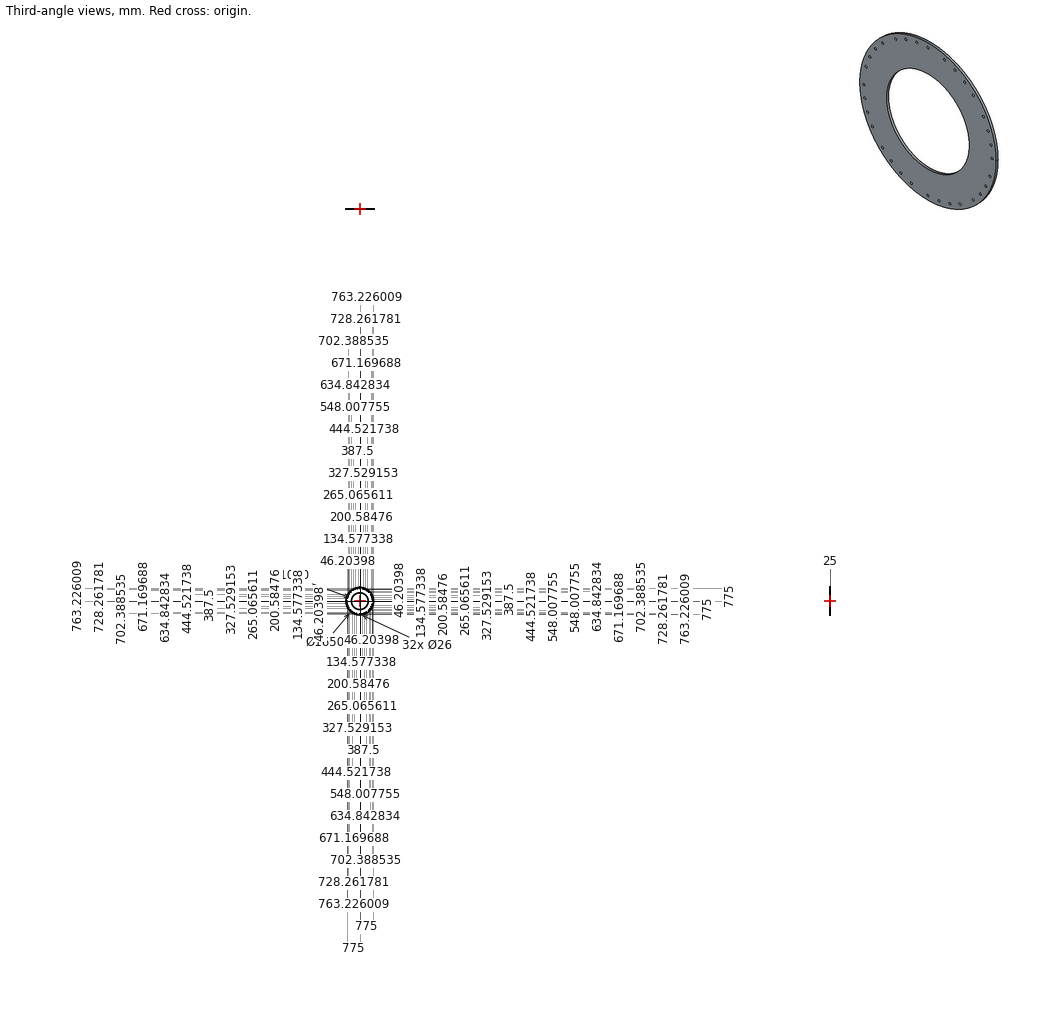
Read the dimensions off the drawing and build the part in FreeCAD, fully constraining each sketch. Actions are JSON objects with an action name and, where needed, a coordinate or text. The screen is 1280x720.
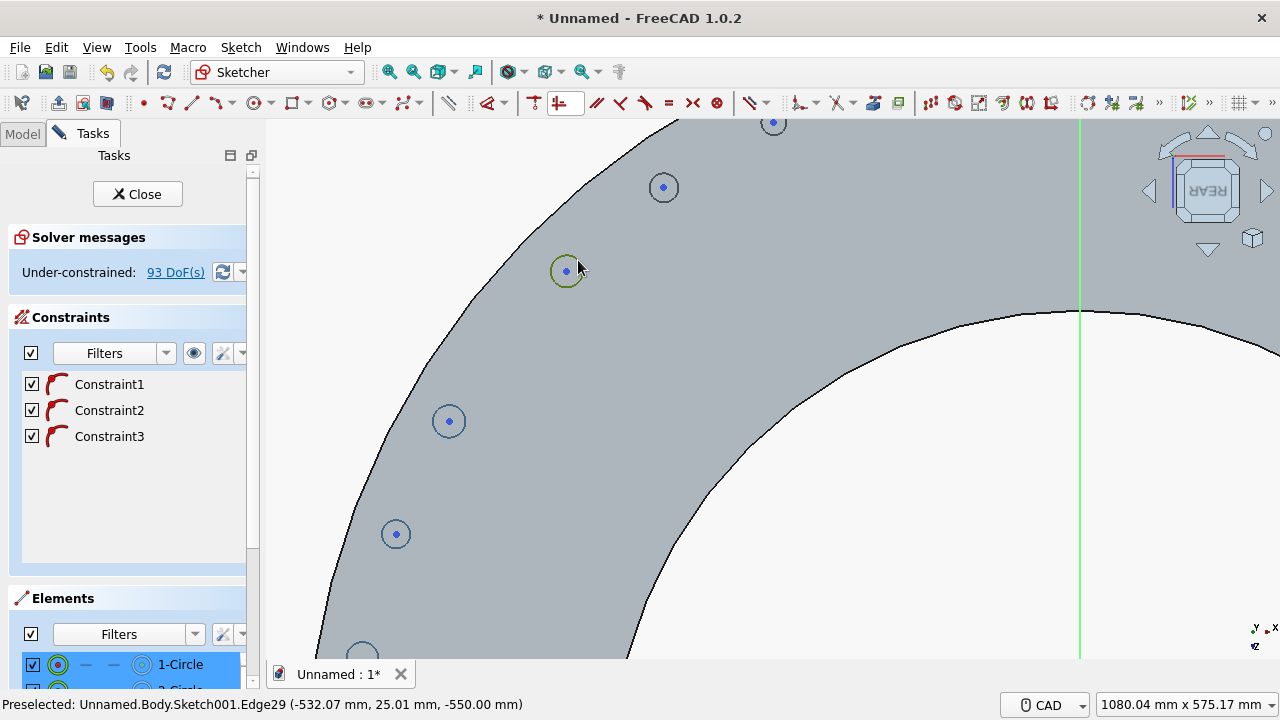
{"action": "left_click", "coordinate": [674, 178]}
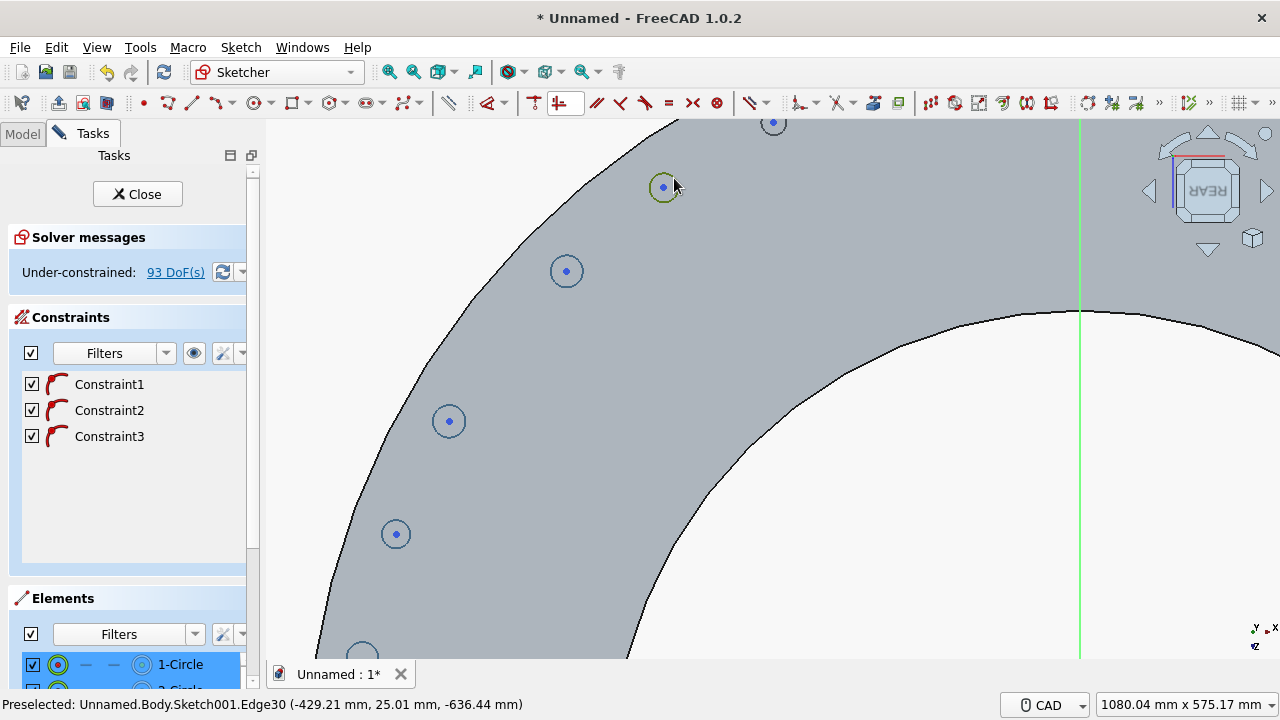
{"action": "scroll", "coordinate": [581, 261], "scroll_direction": "down", "scroll_amount": 7}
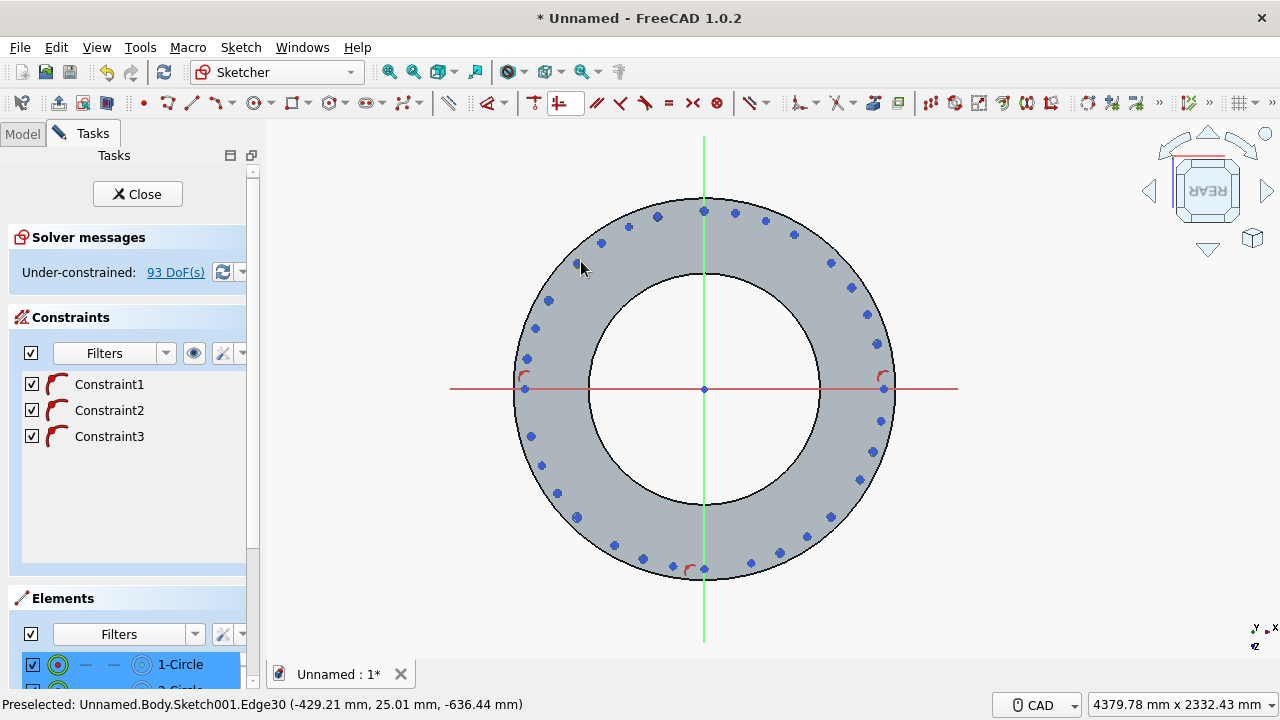
{"action": "scroll", "coordinate": [631, 225], "scroll_direction": "up", "scroll_amount": 8}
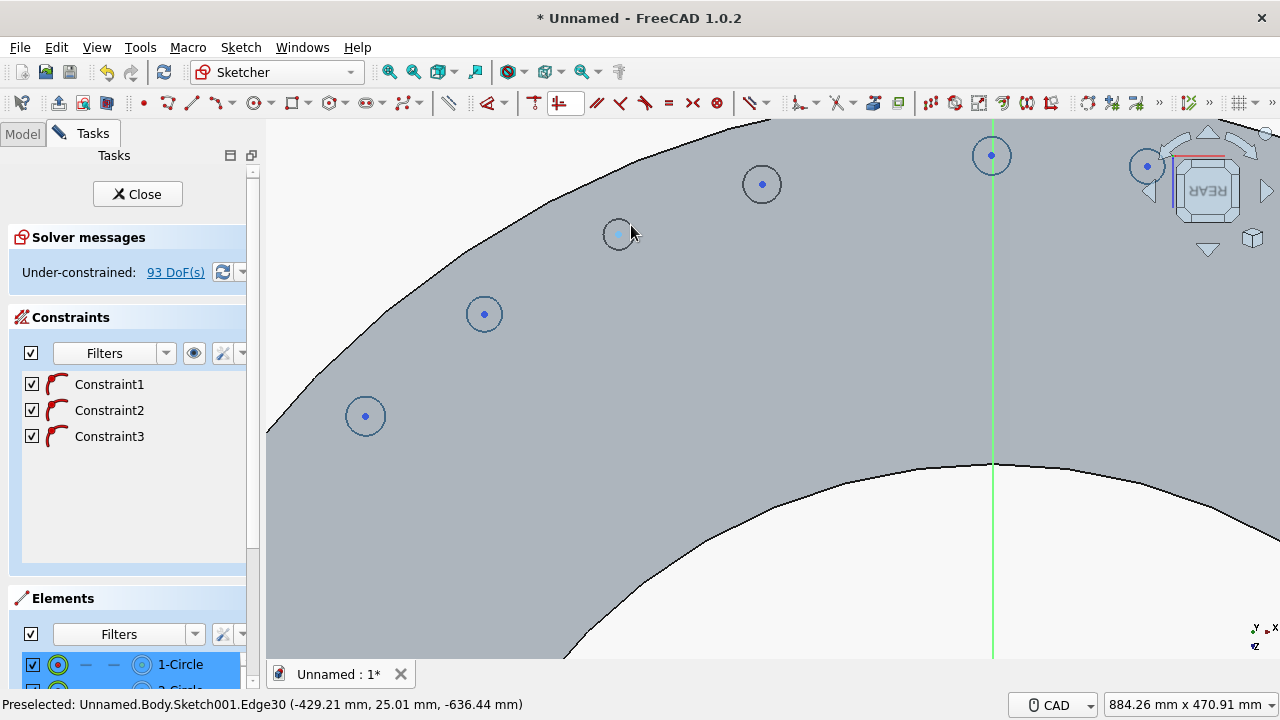
{"action": "left_click", "coordinate": [630, 224]}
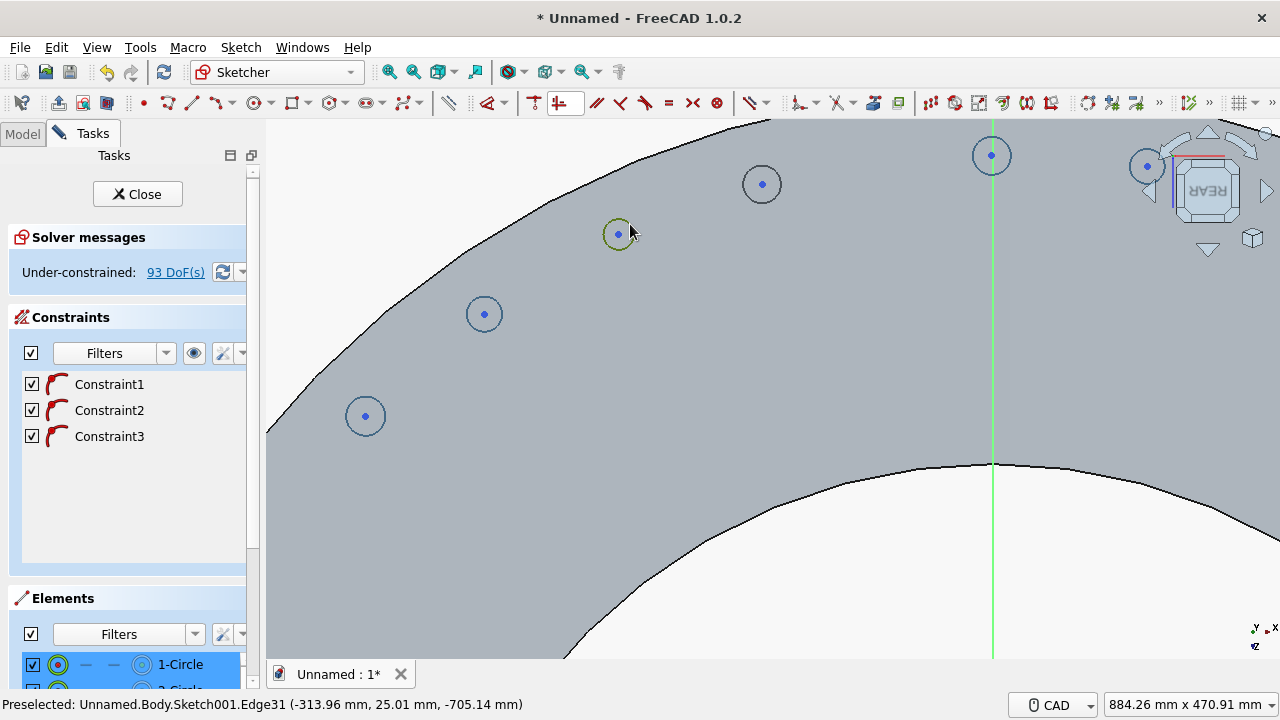
{"action": "left_click", "coordinate": [775, 171]}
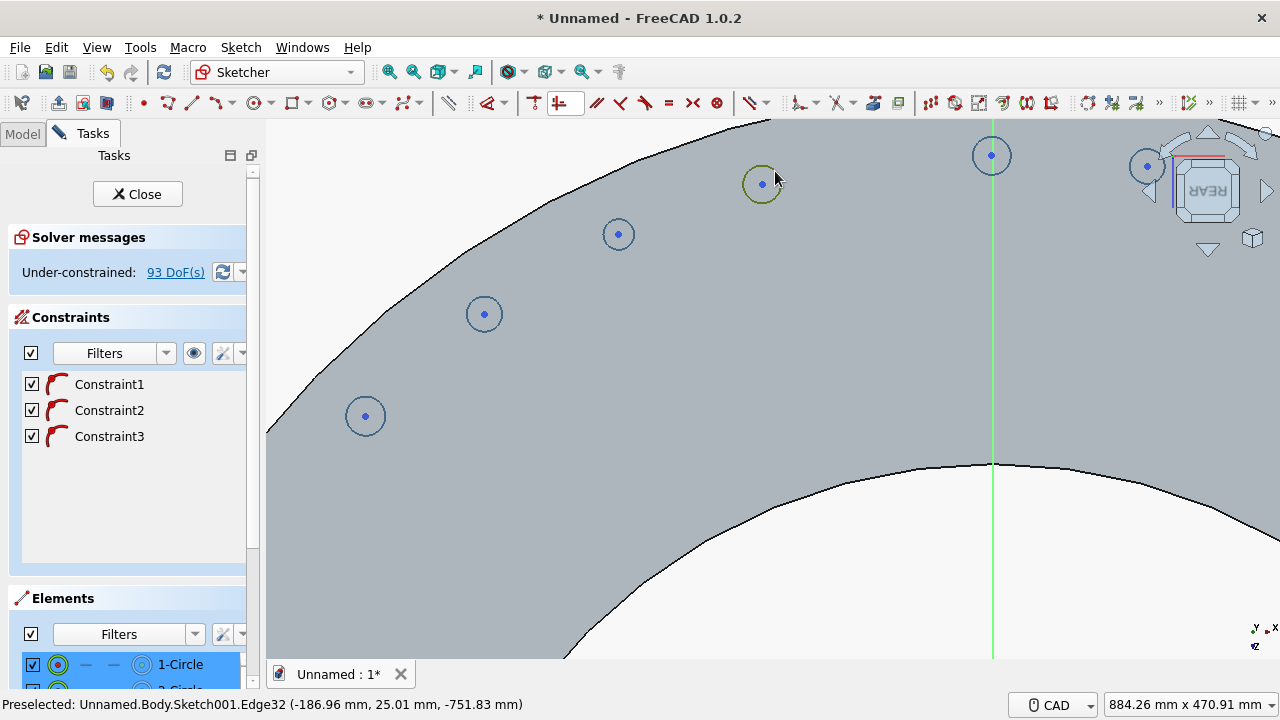
{"action": "key", "text": "e"}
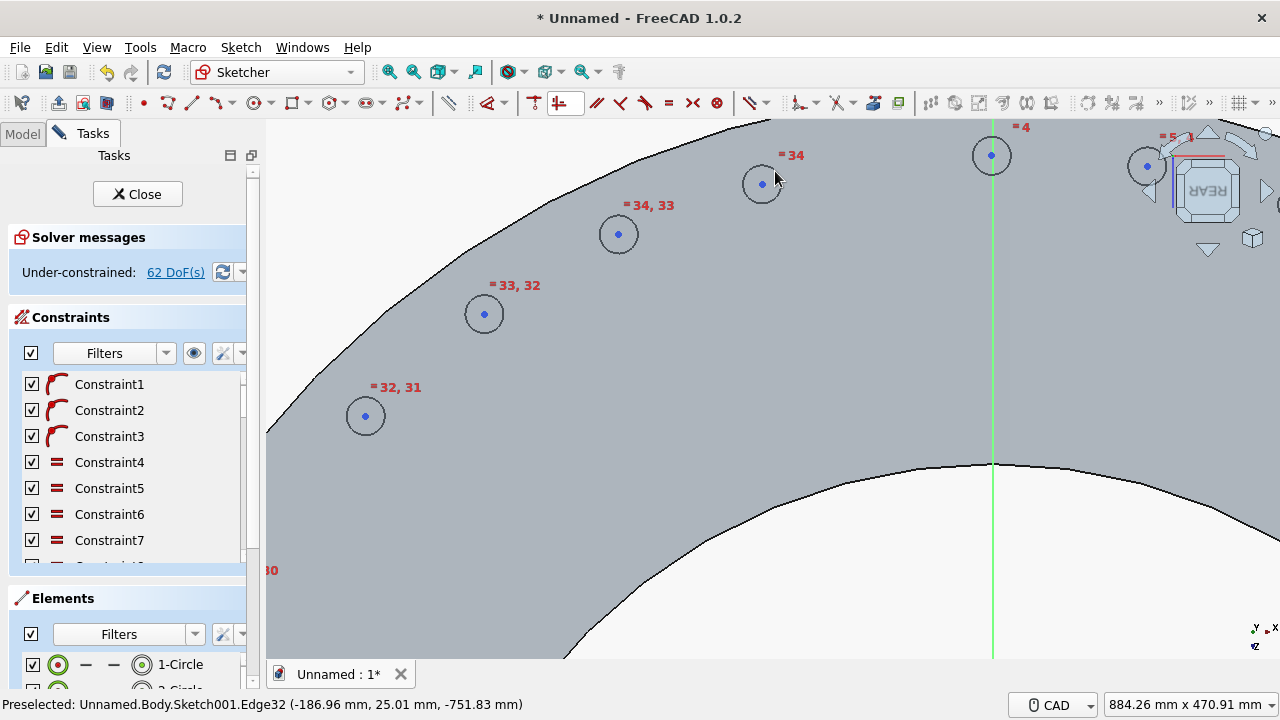
{"action": "scroll", "coordinate": [632, 225], "scroll_direction": "down", "scroll_amount": 8}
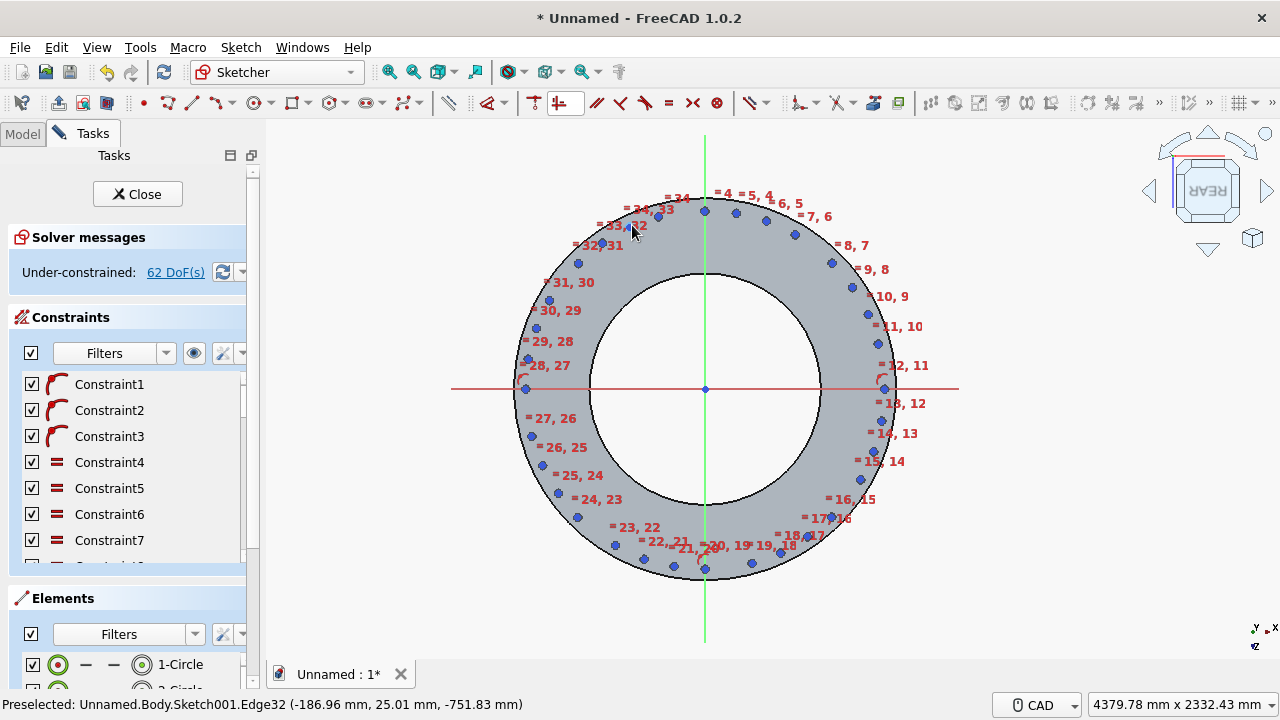
{"action": "left_click", "coordinate": [705, 211]}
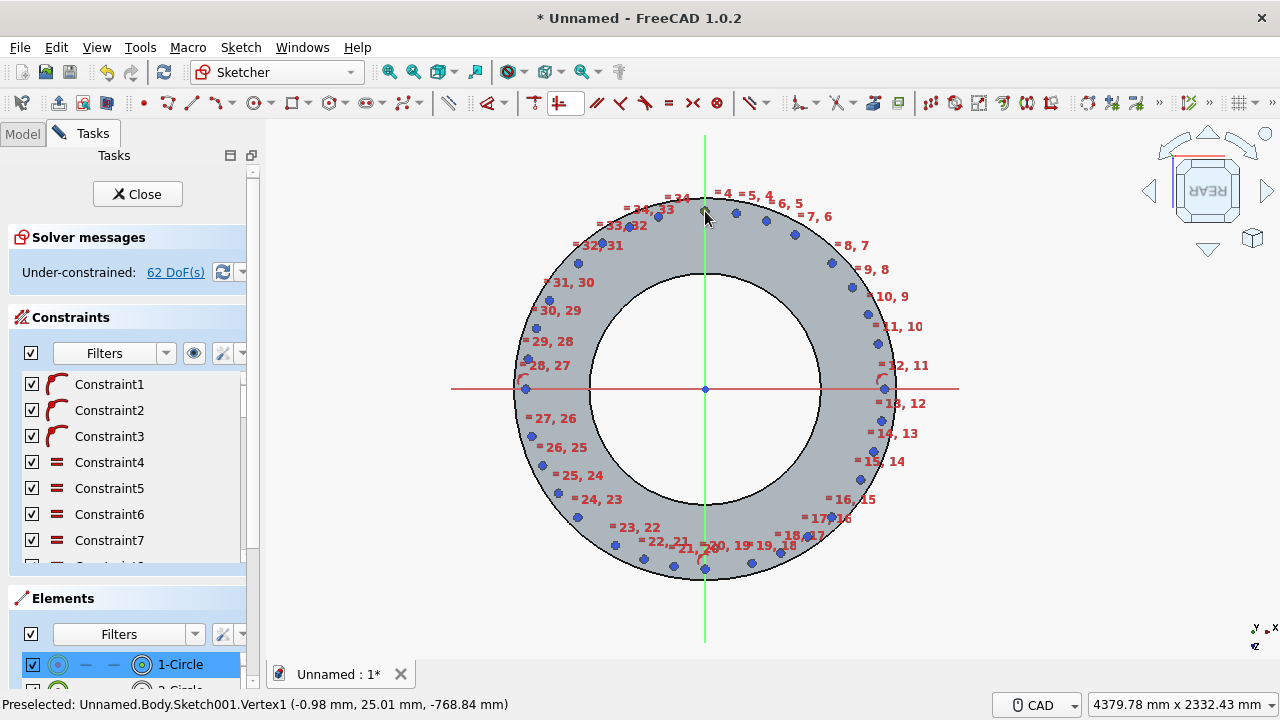
{"action": "left_click", "coordinate": [705, 527]}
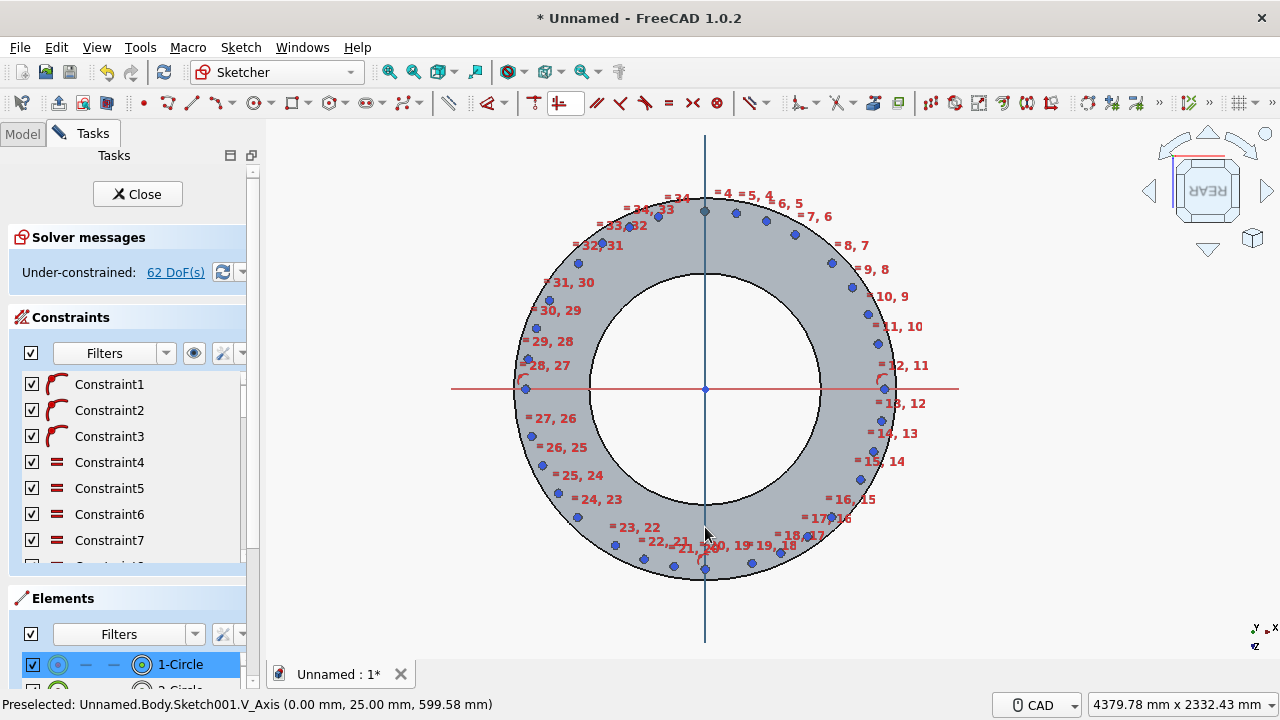
{"action": "left_click", "coordinate": [534, 104]}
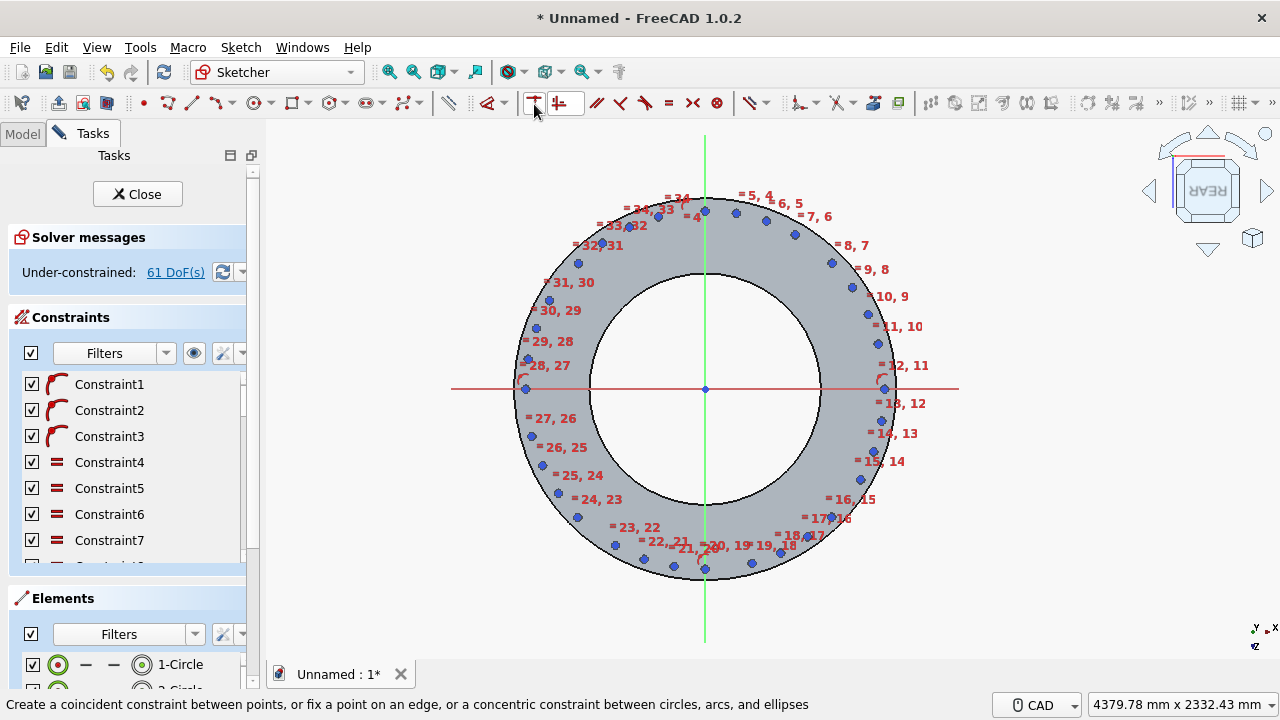
{"action": "scroll", "coordinate": [702, 208], "scroll_direction": "up", "scroll_amount": 10}